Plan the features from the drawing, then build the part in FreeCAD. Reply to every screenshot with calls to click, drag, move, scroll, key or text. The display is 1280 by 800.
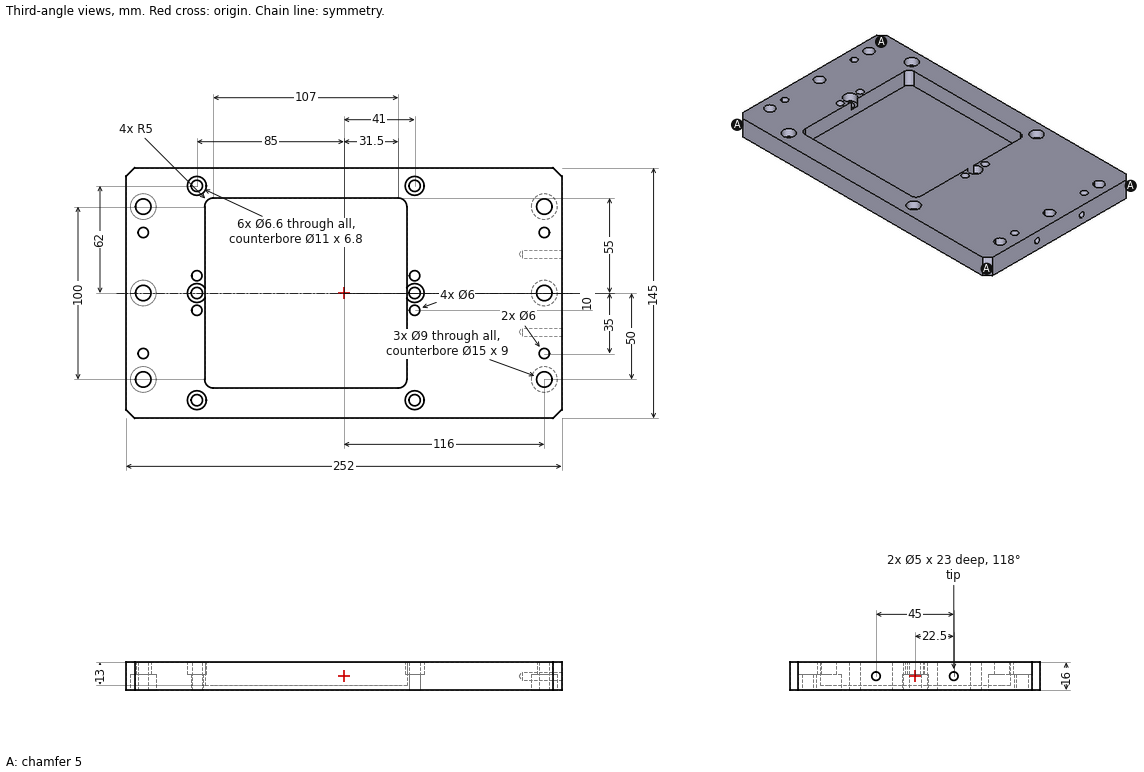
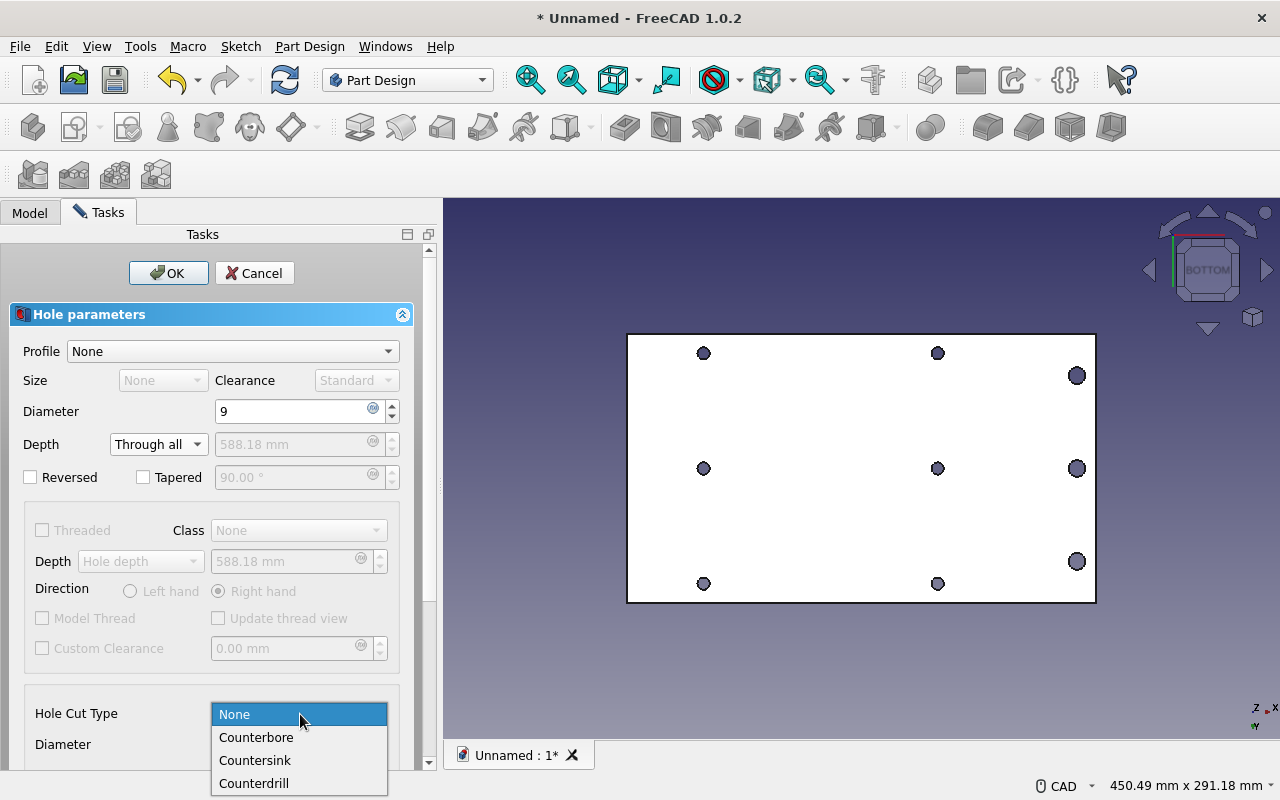
click(298, 738)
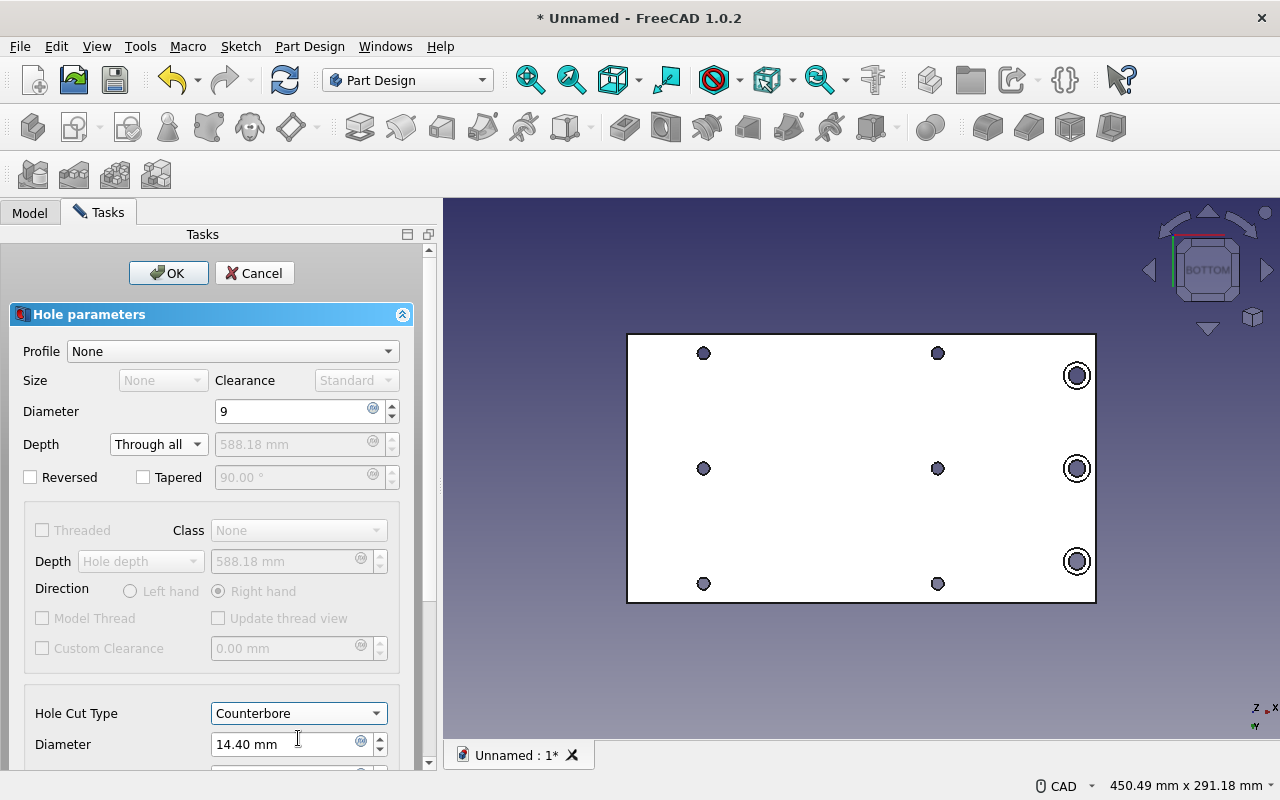
triple_click(292, 744)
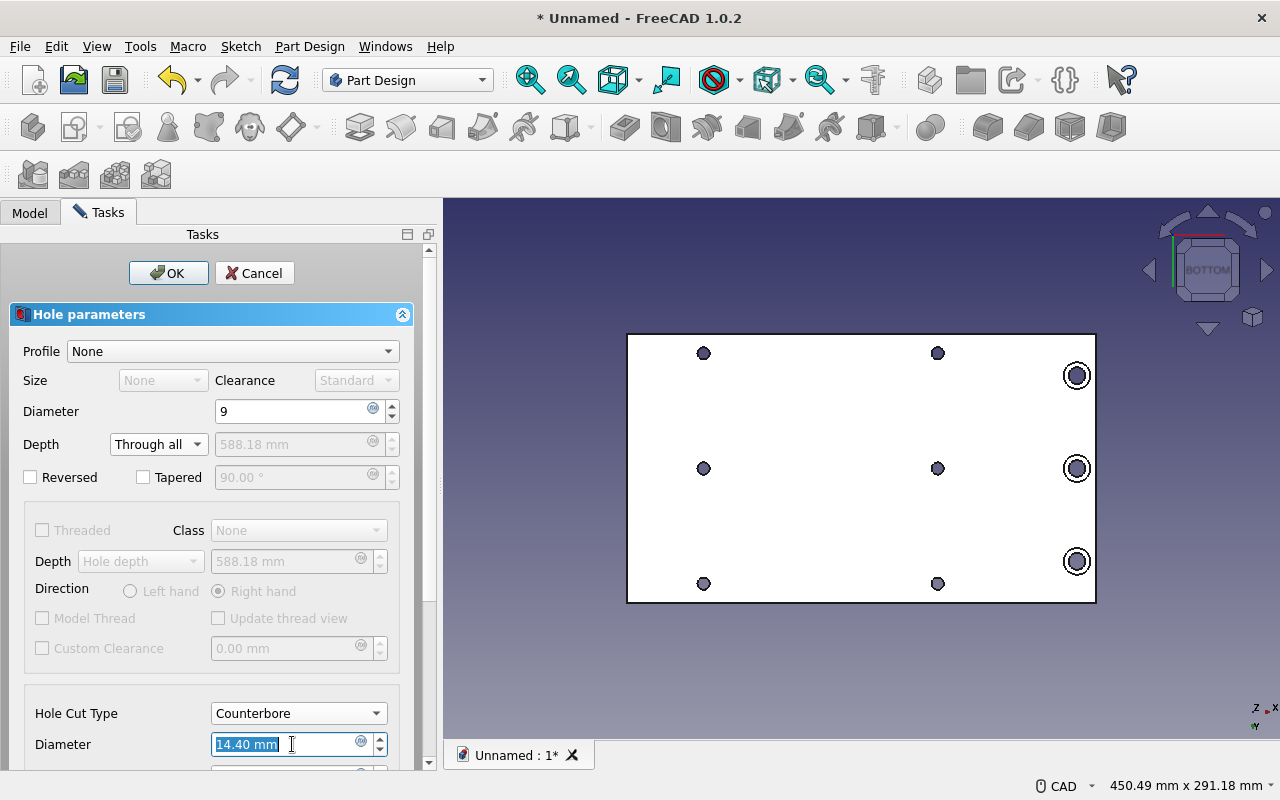
text(15)
key(Tab)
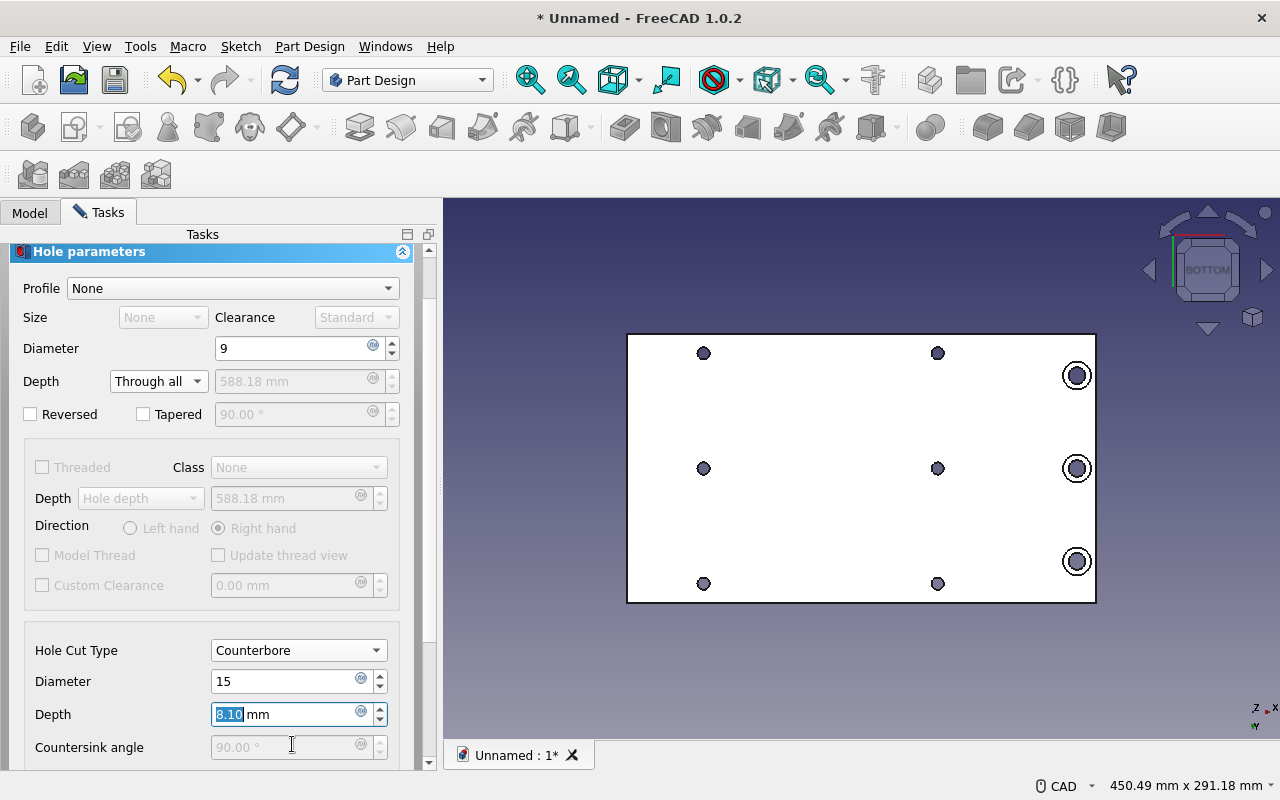
text(9)
key(Tab)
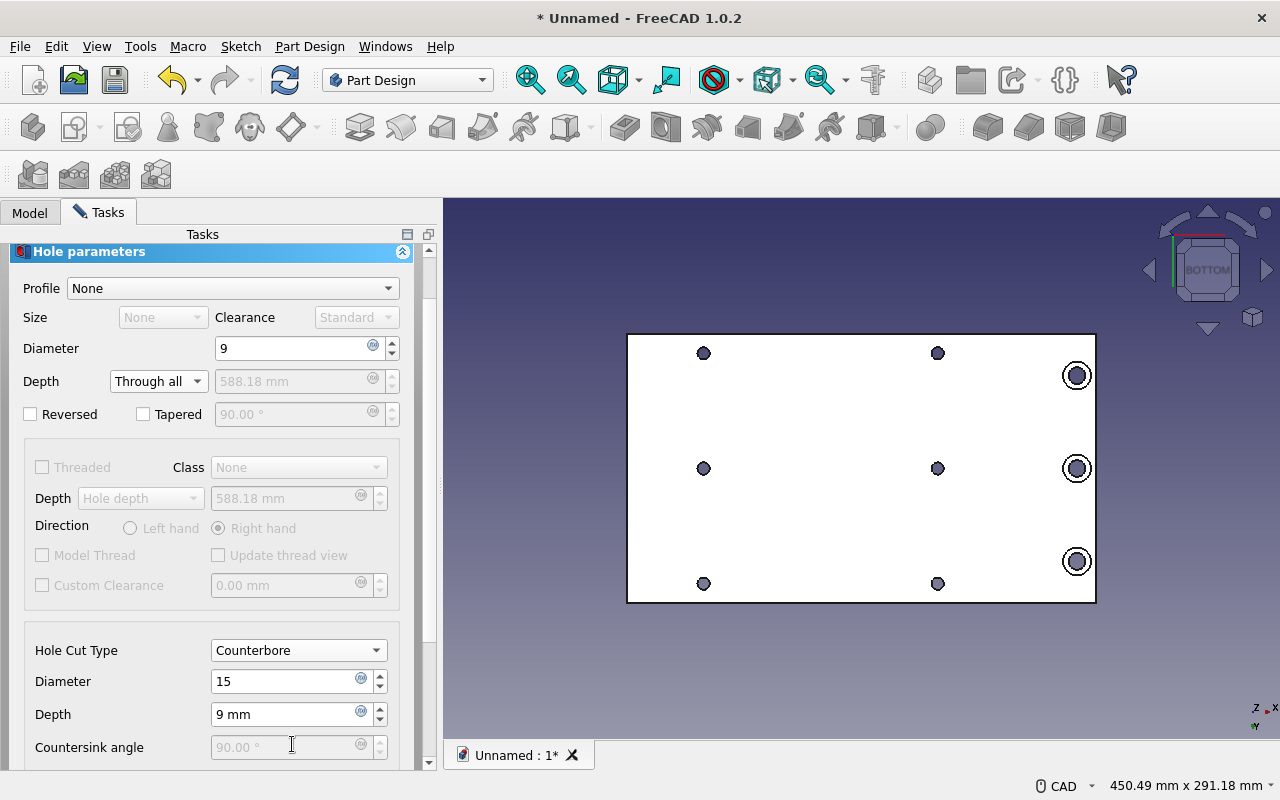
scroll(429, 507, up, 2)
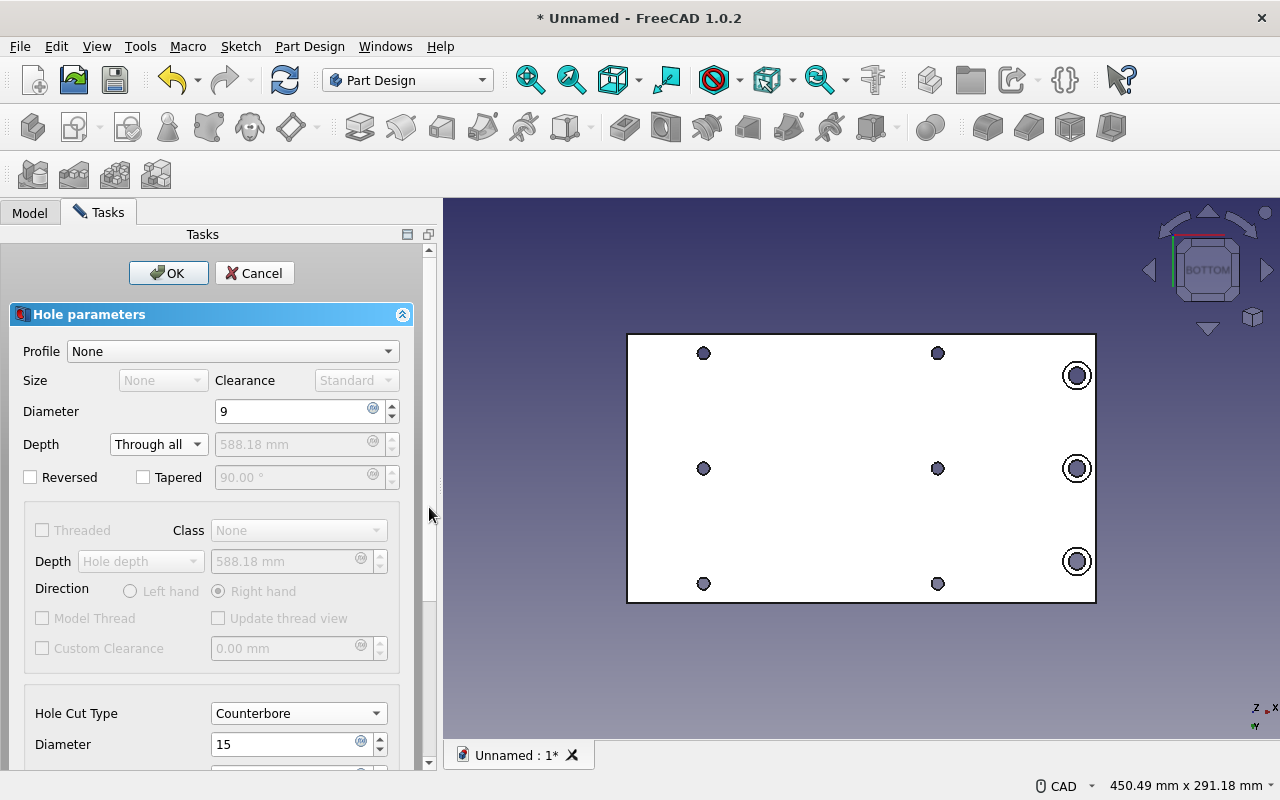
click(169, 273)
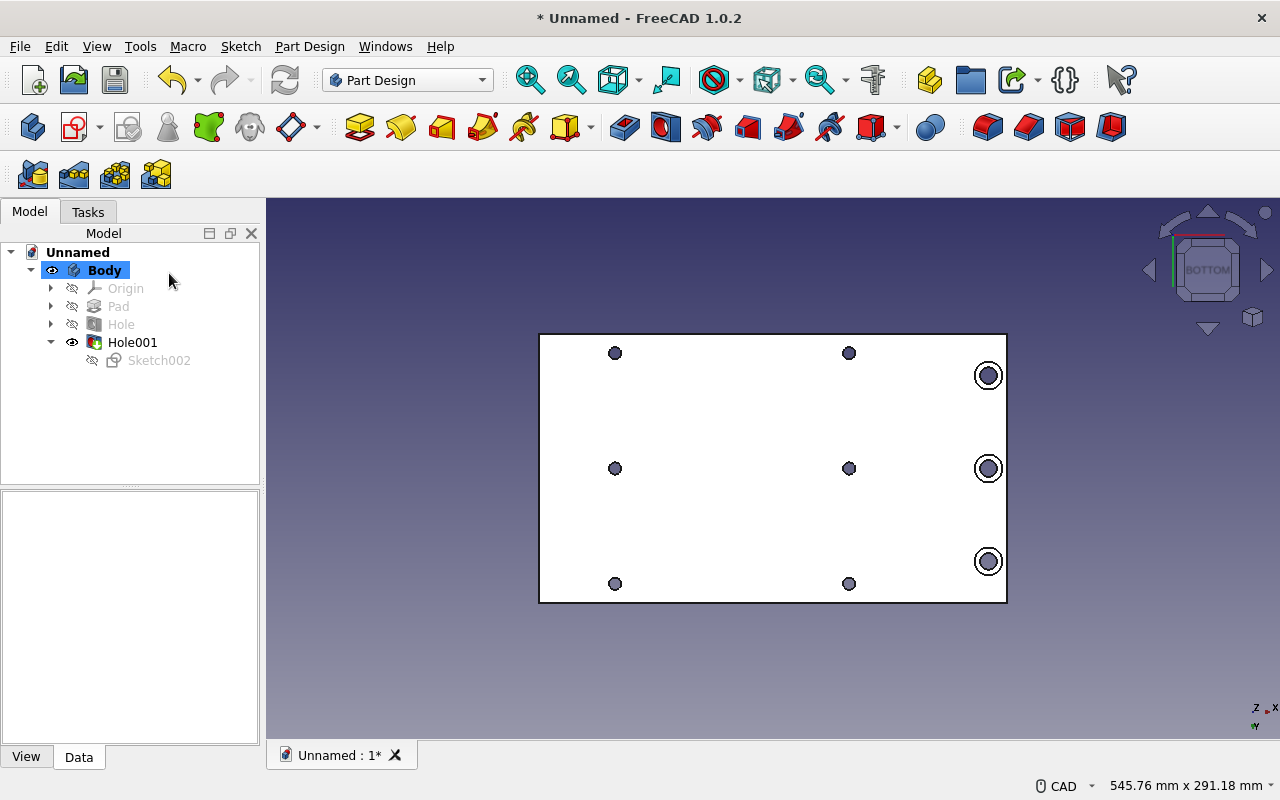
click(706, 429)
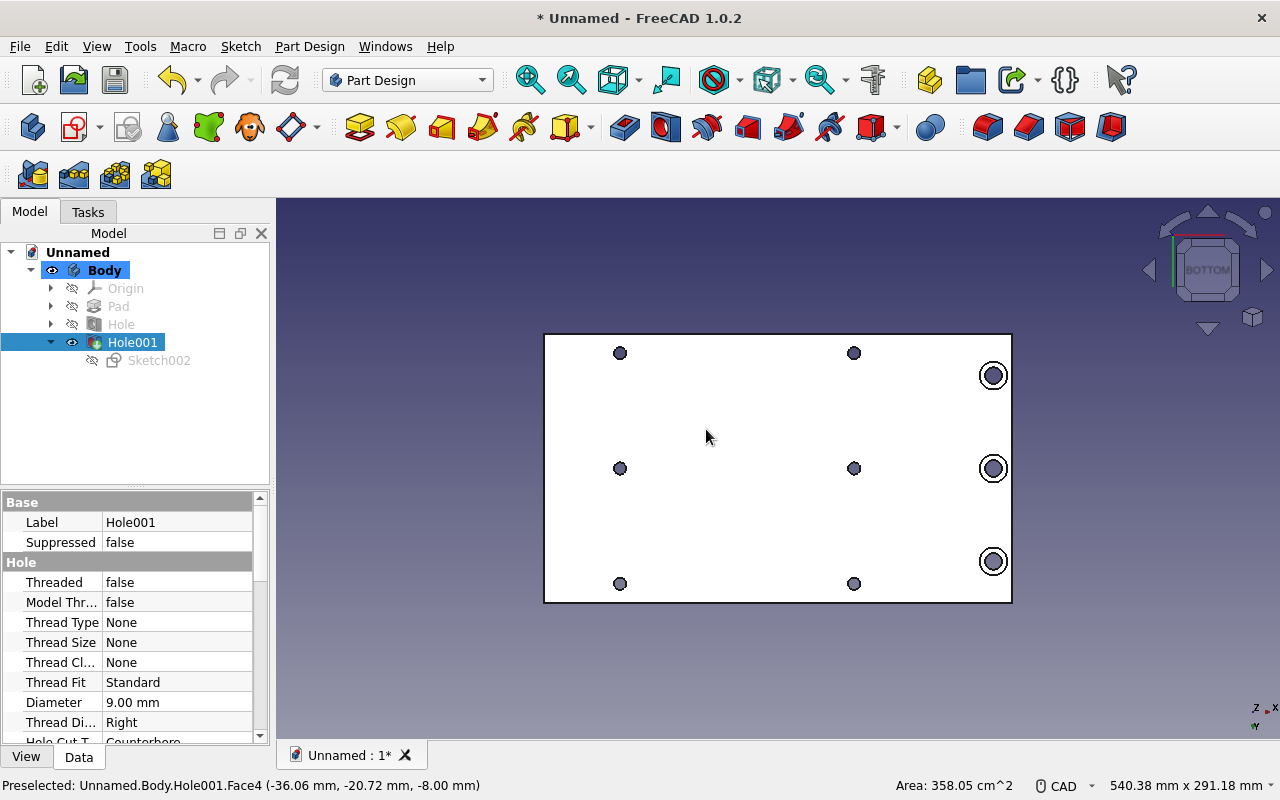
click(74, 128)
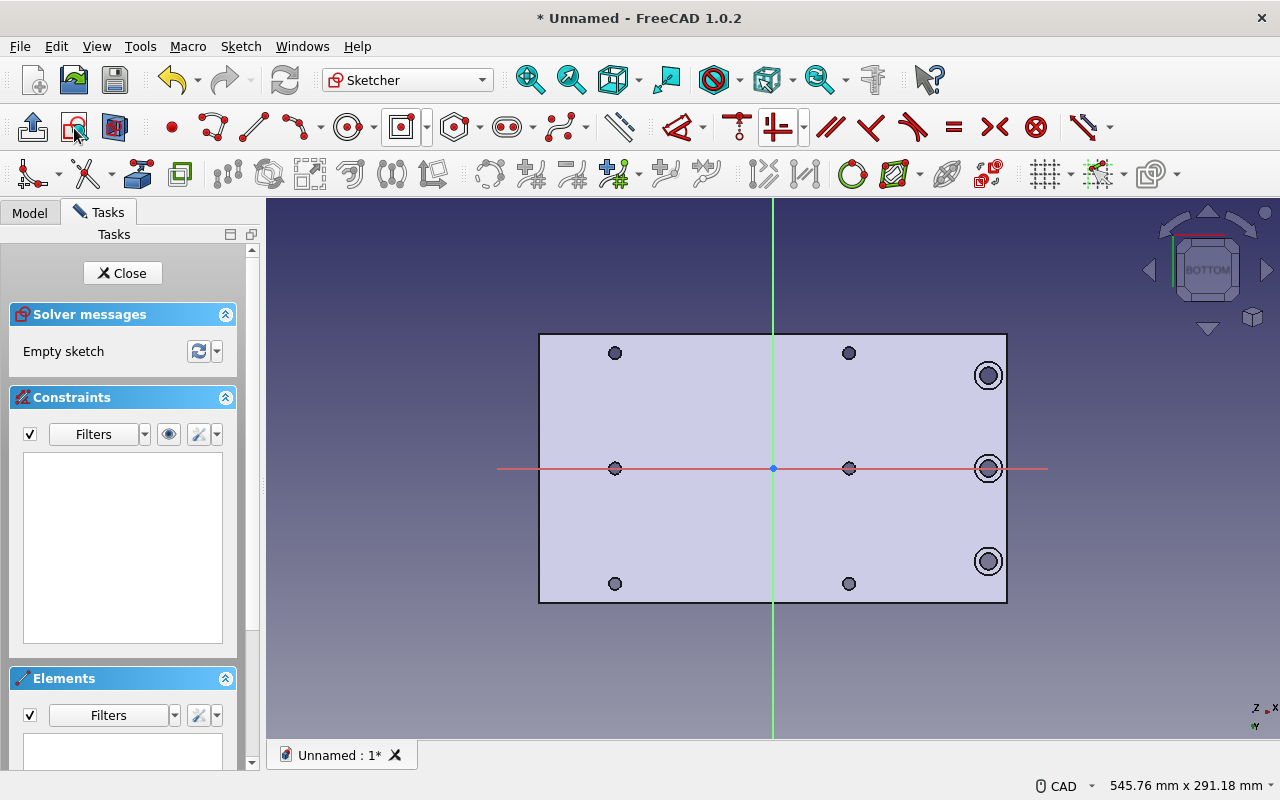
scroll(1030, 469, up, 4)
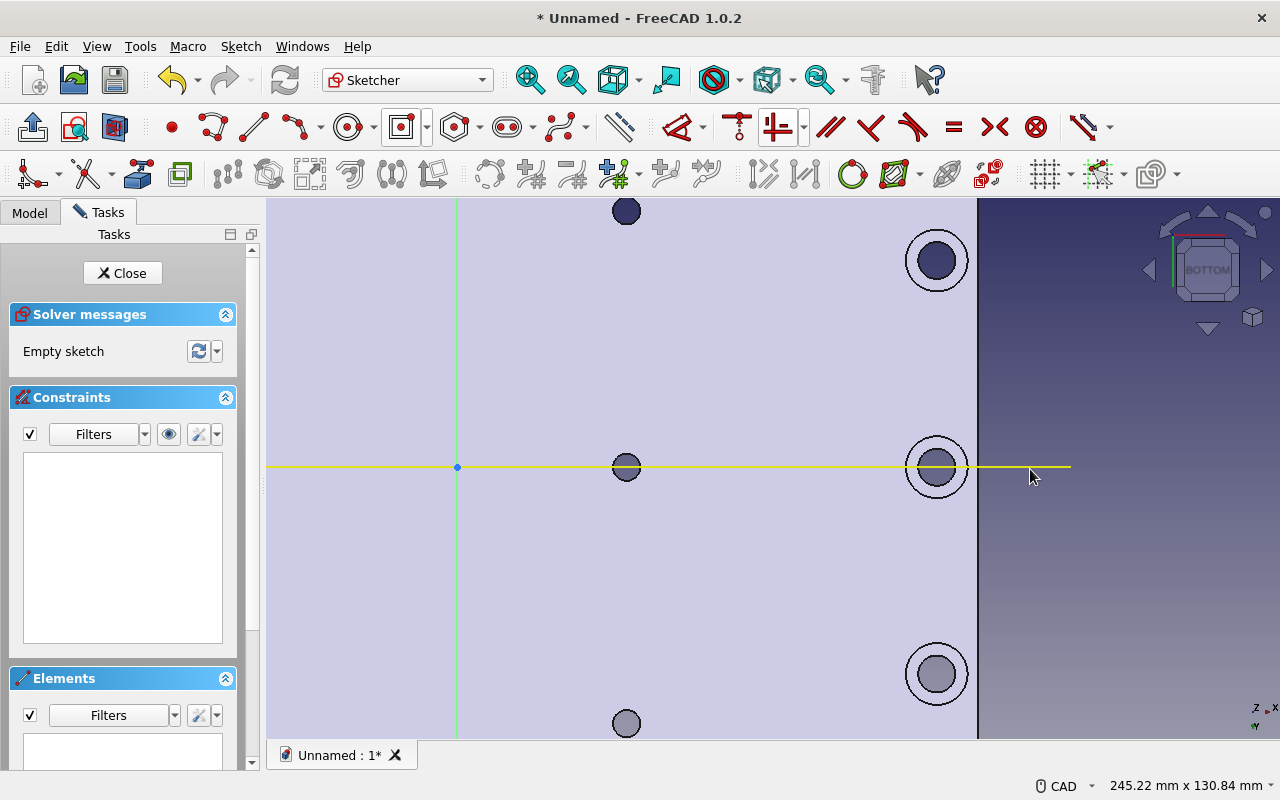
key(g)
key(c)